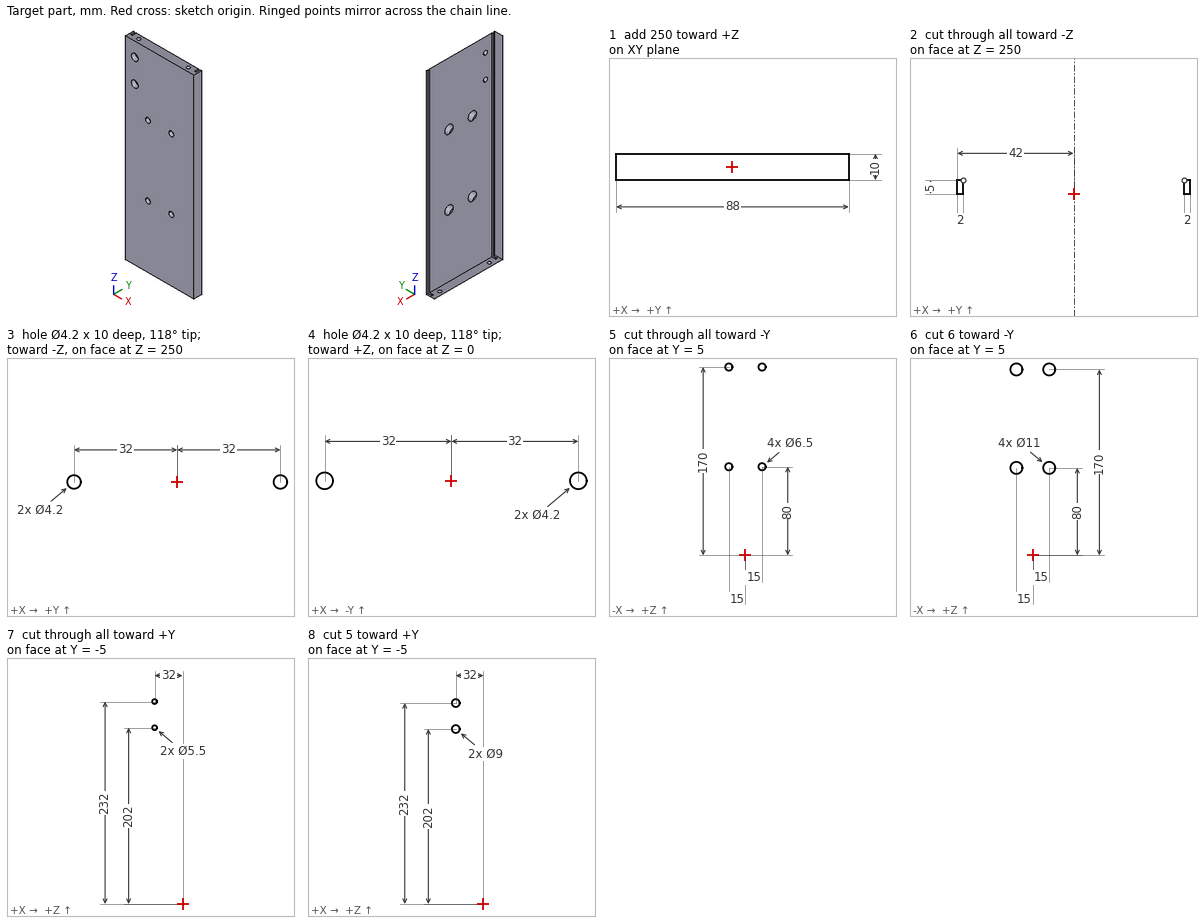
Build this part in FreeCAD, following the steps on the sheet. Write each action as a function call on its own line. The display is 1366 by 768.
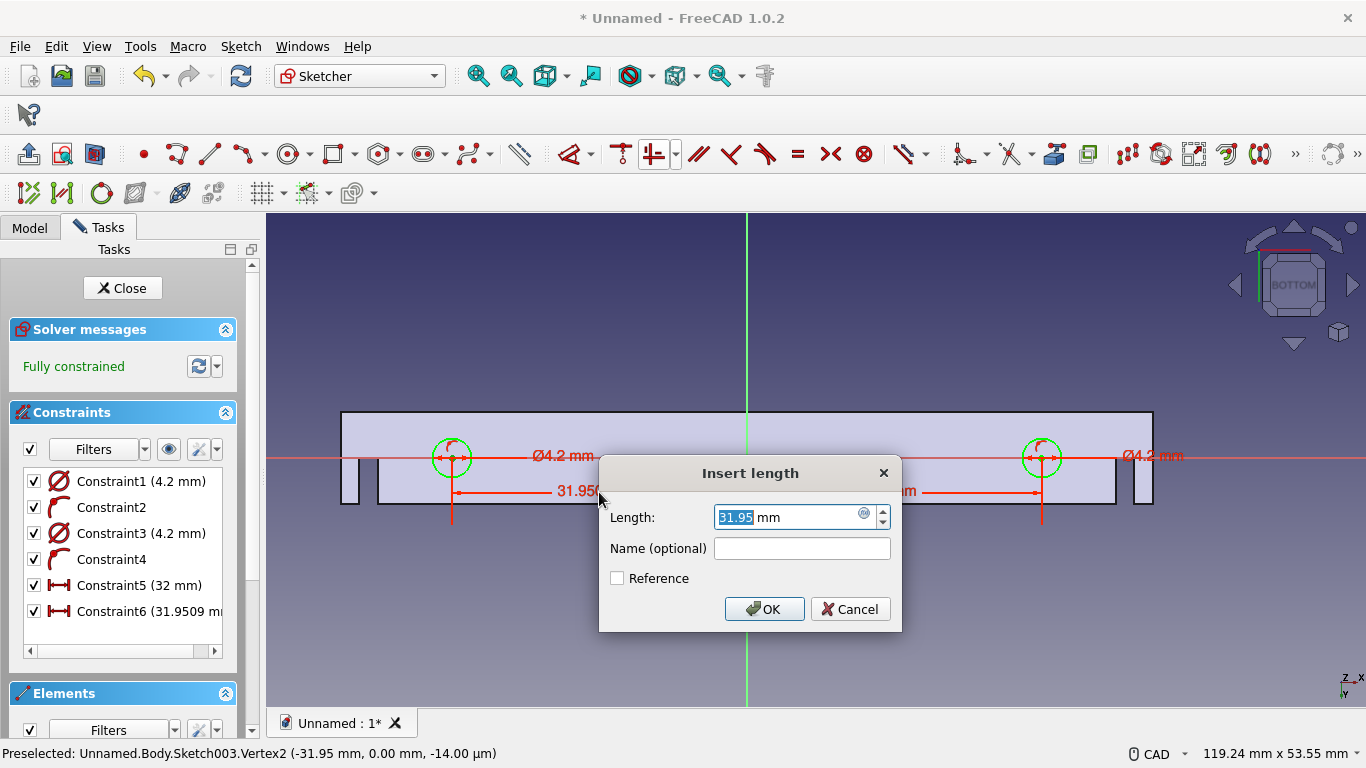
text(32)
key(Return)
key(Escape)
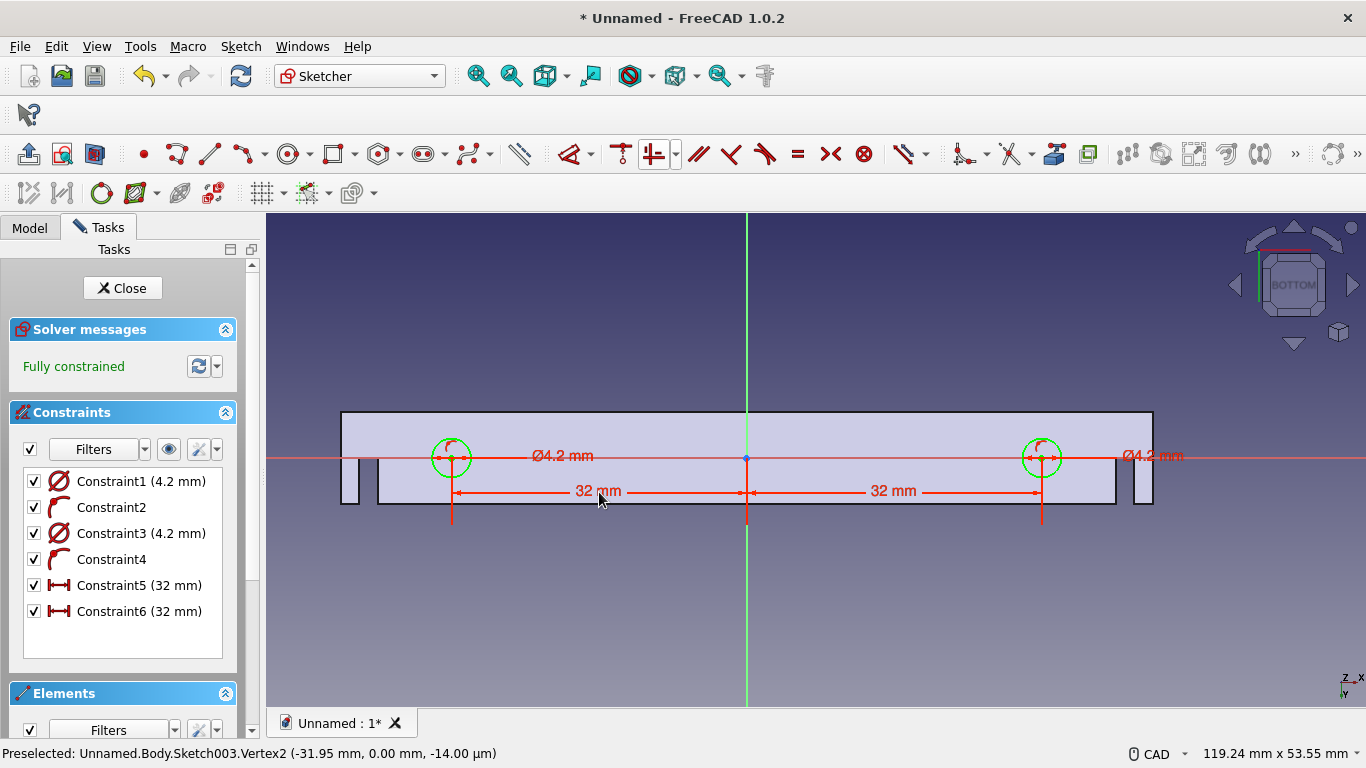
click(123, 288)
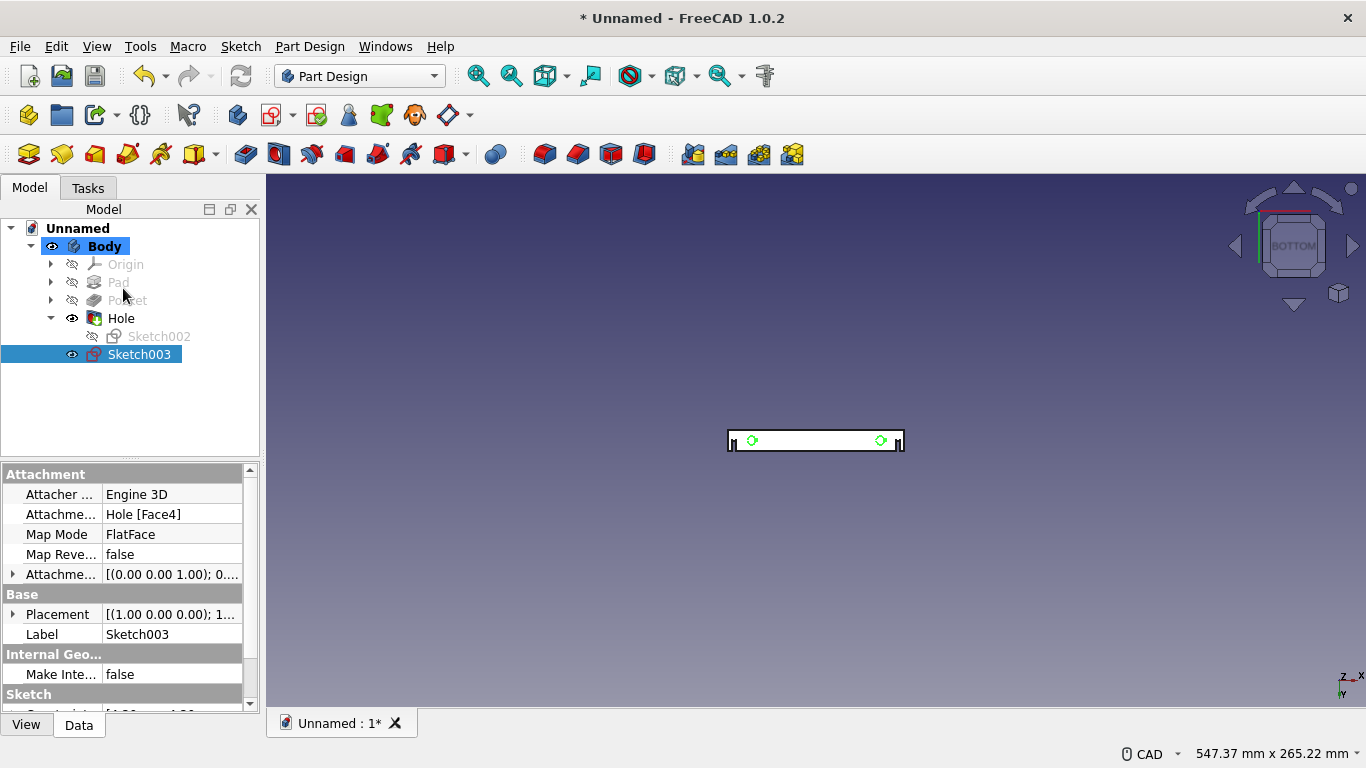
click(279, 154)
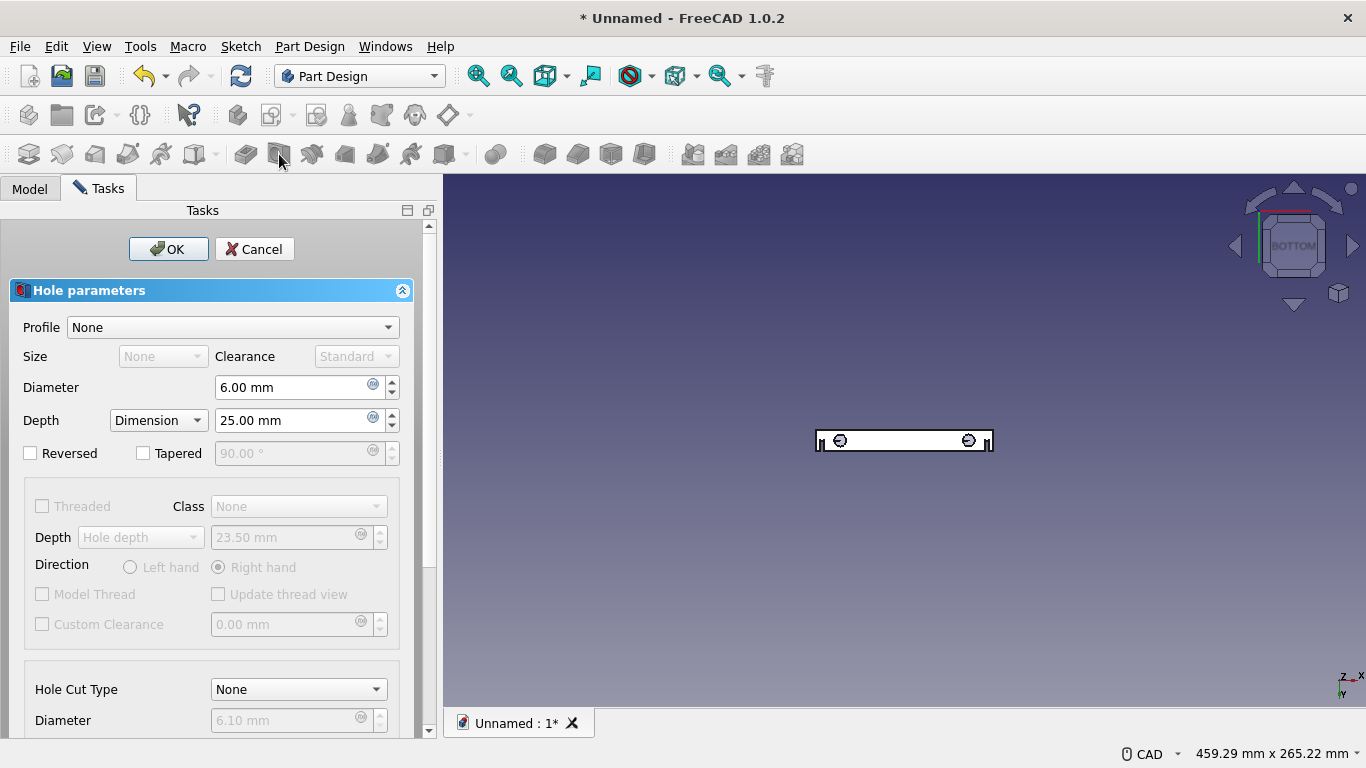
triple_click(300, 388)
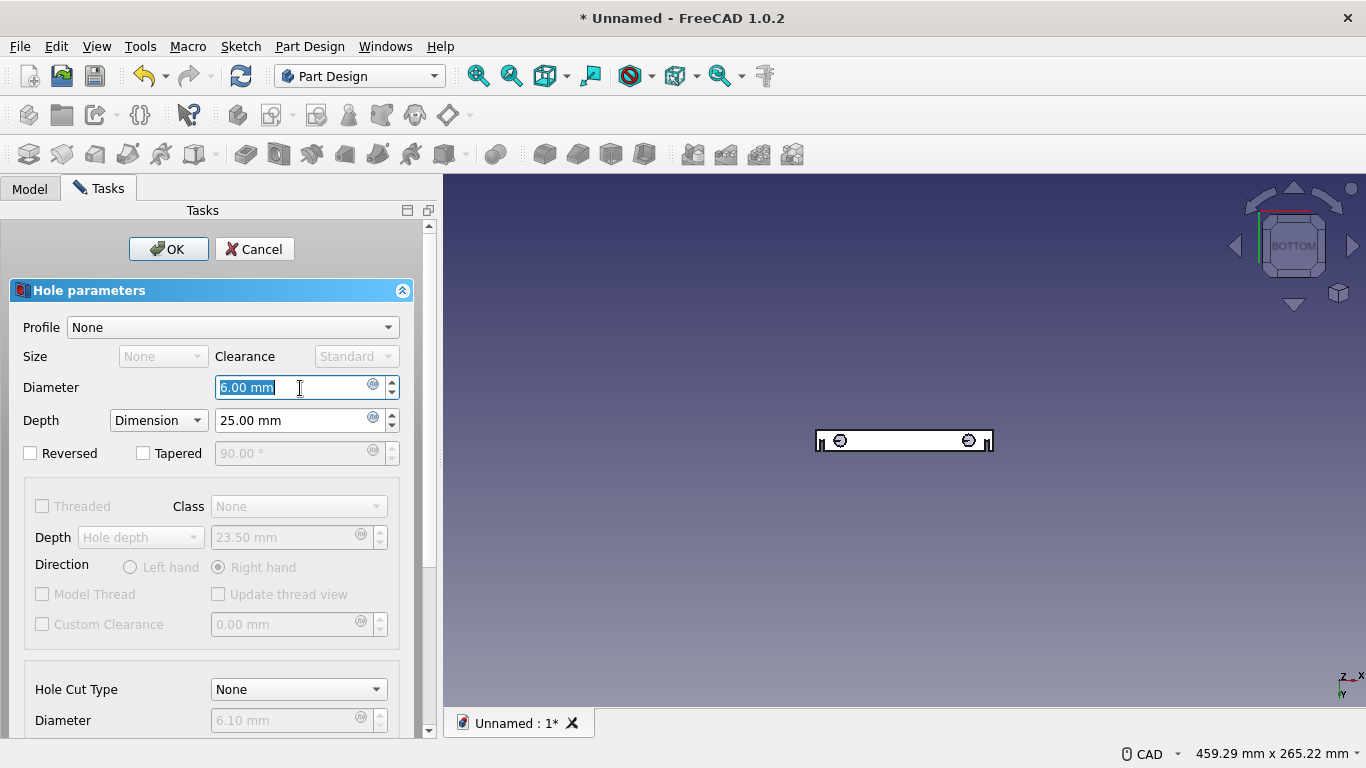
text(4.2)
key(Tab)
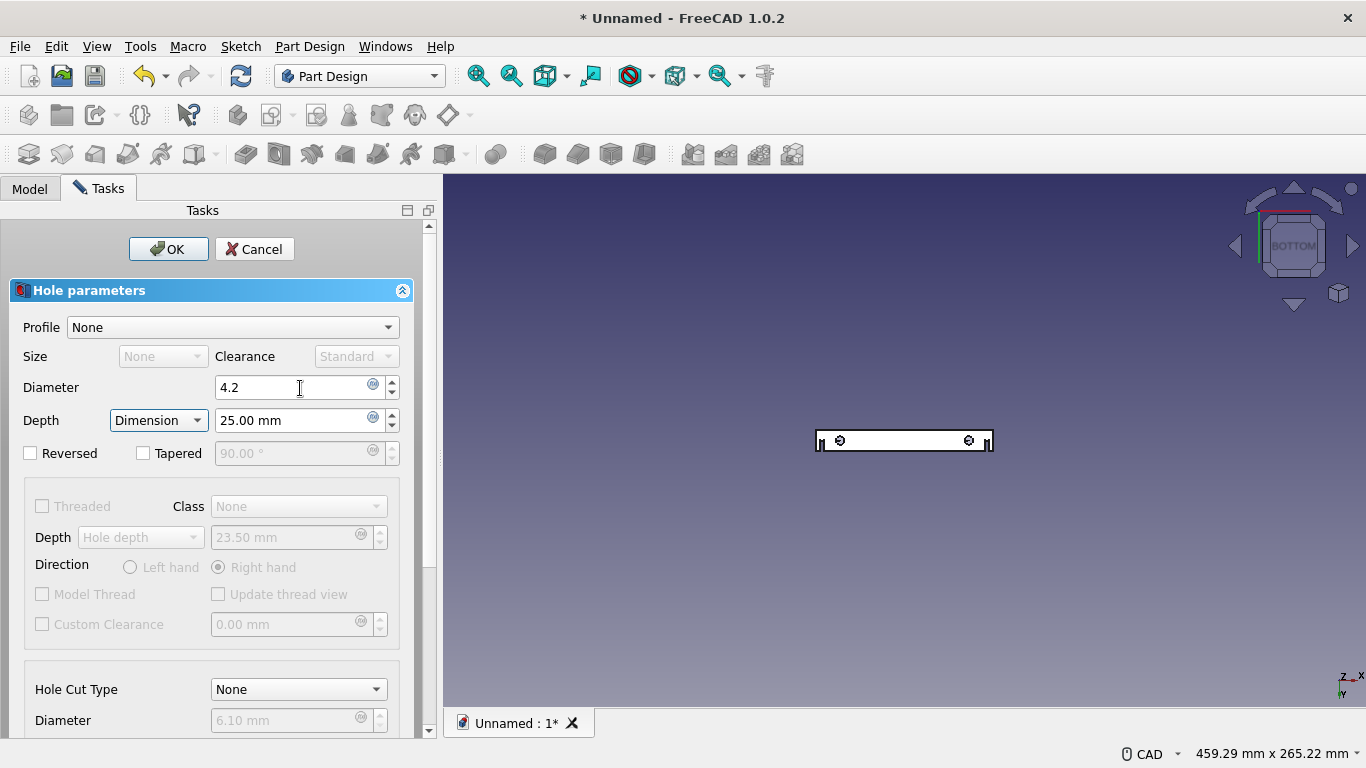
triple_click(300, 420)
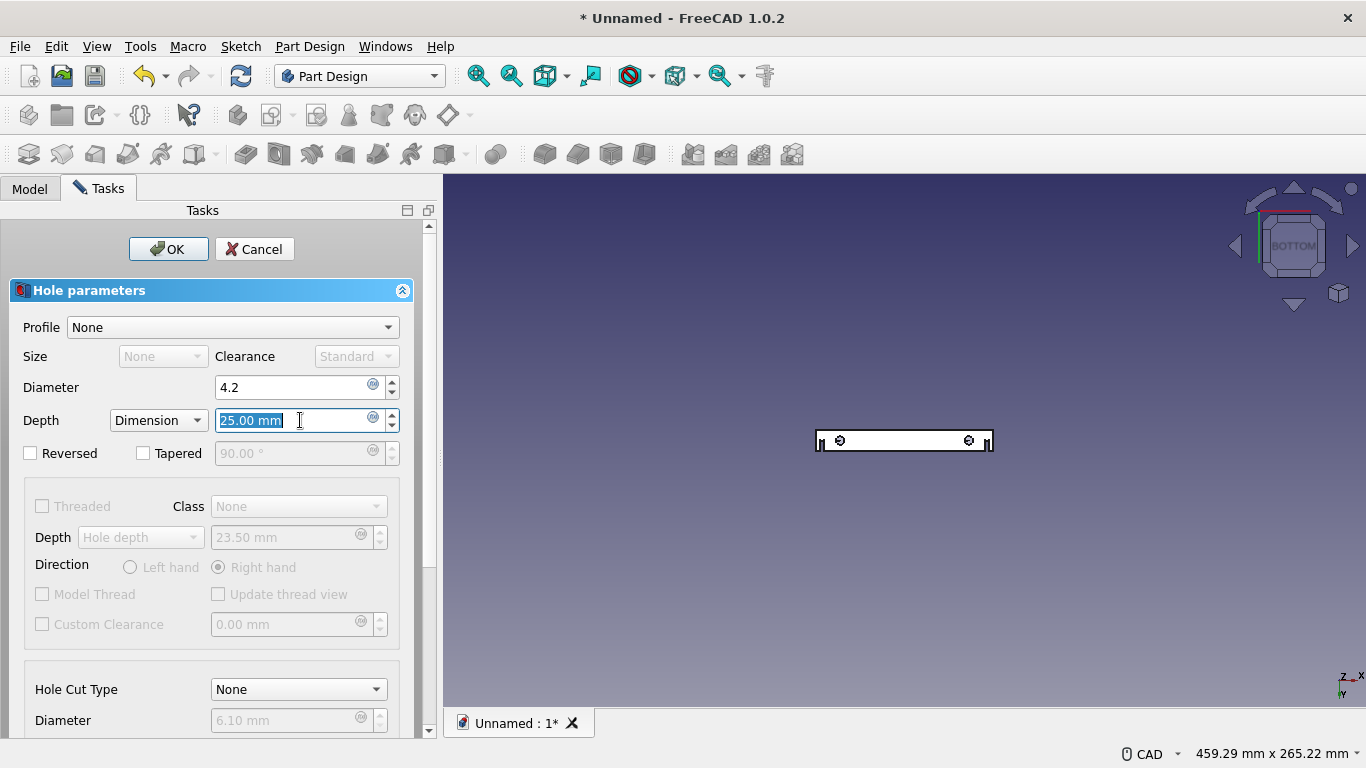
text(10)
key(Tab)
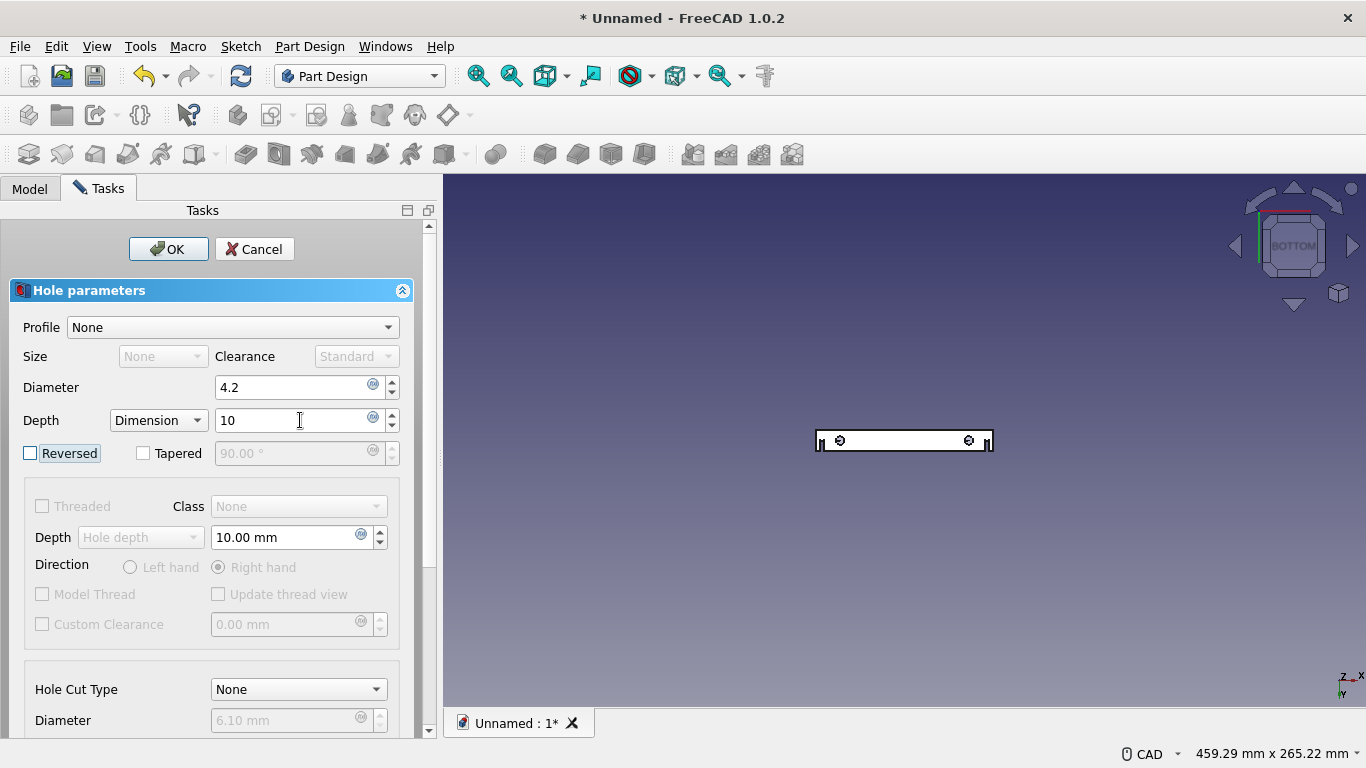
click(169, 249)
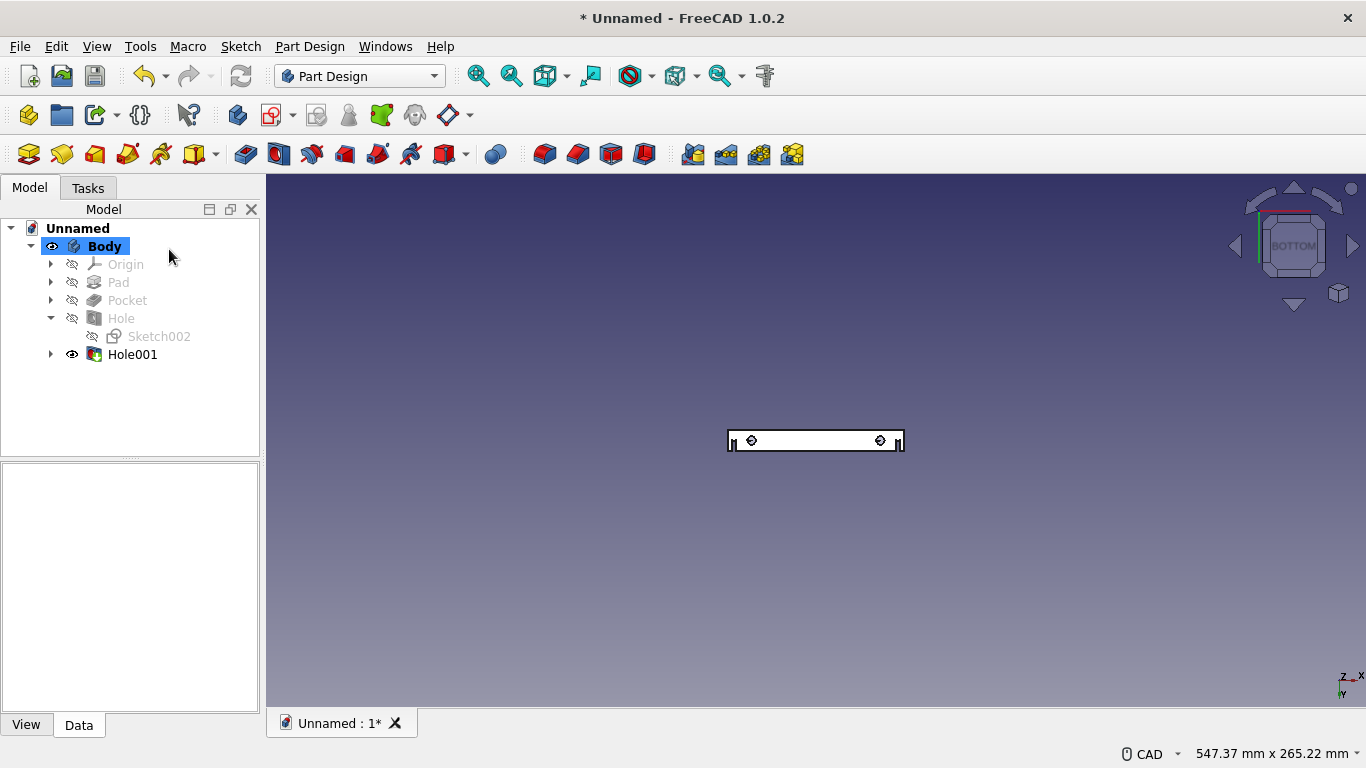
key(v)
key(f)